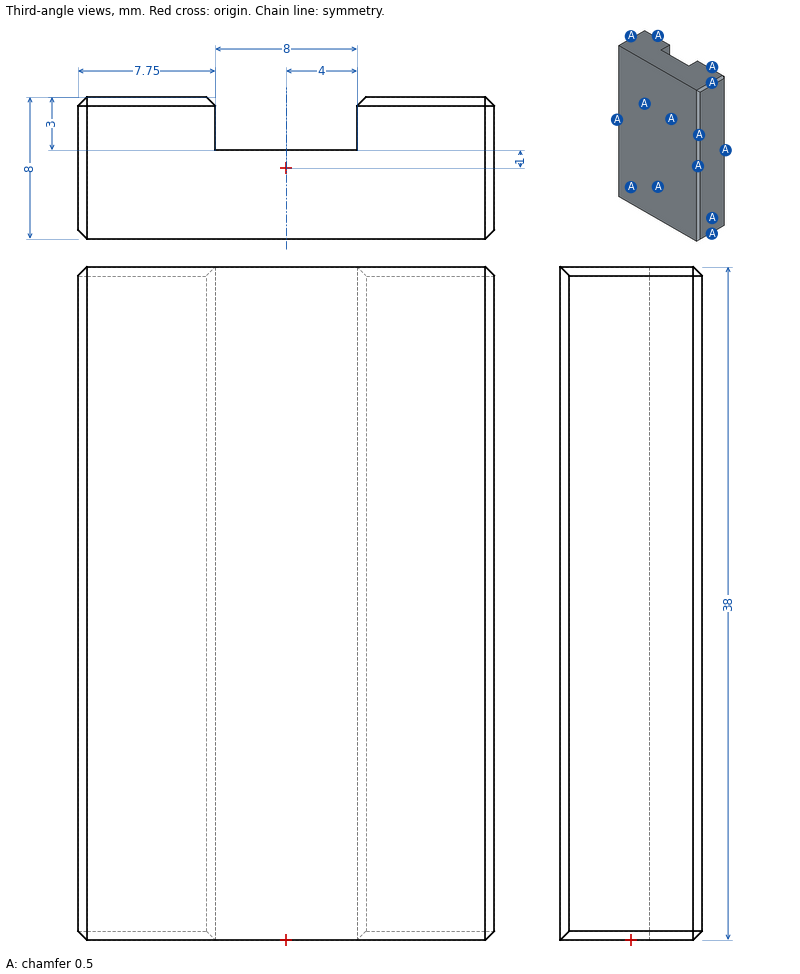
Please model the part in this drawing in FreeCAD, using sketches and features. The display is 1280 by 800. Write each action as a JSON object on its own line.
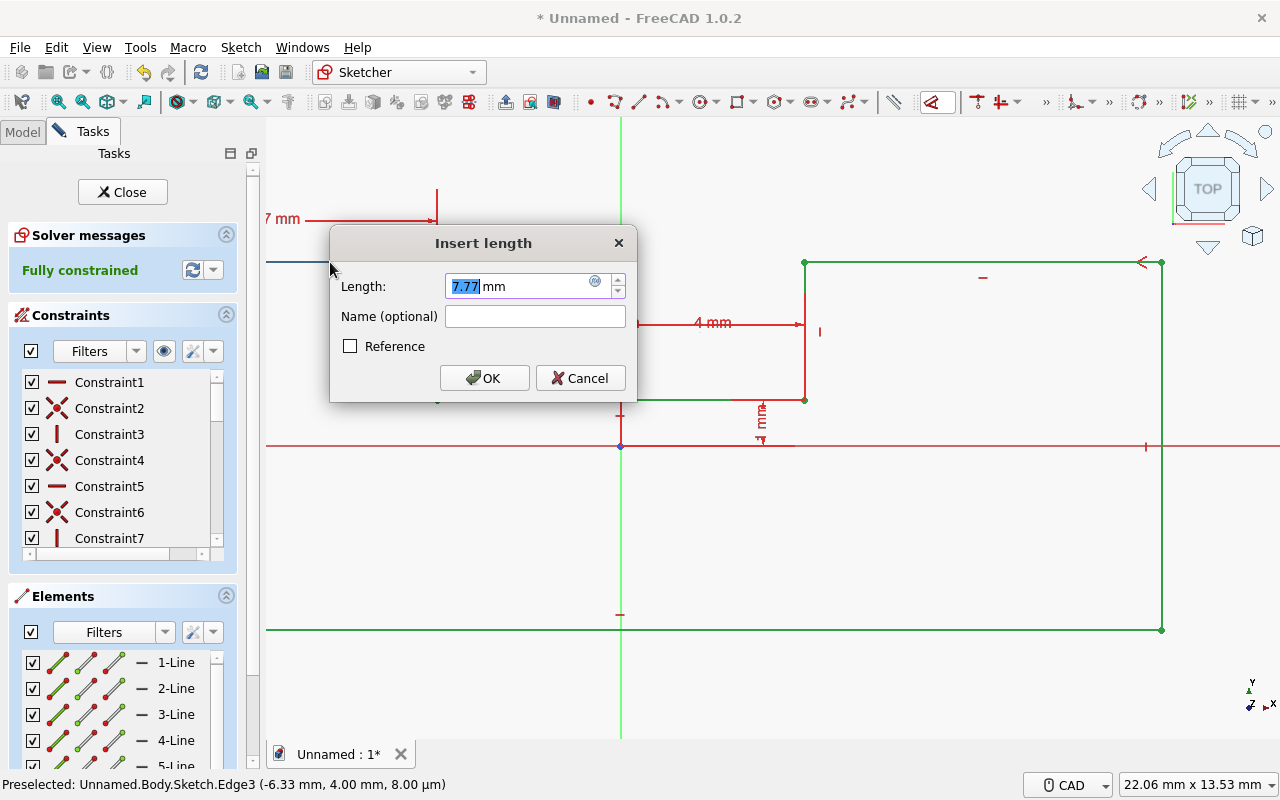
{"action": "type", "text": "7.75"}
{"action": "key", "text": "Return"}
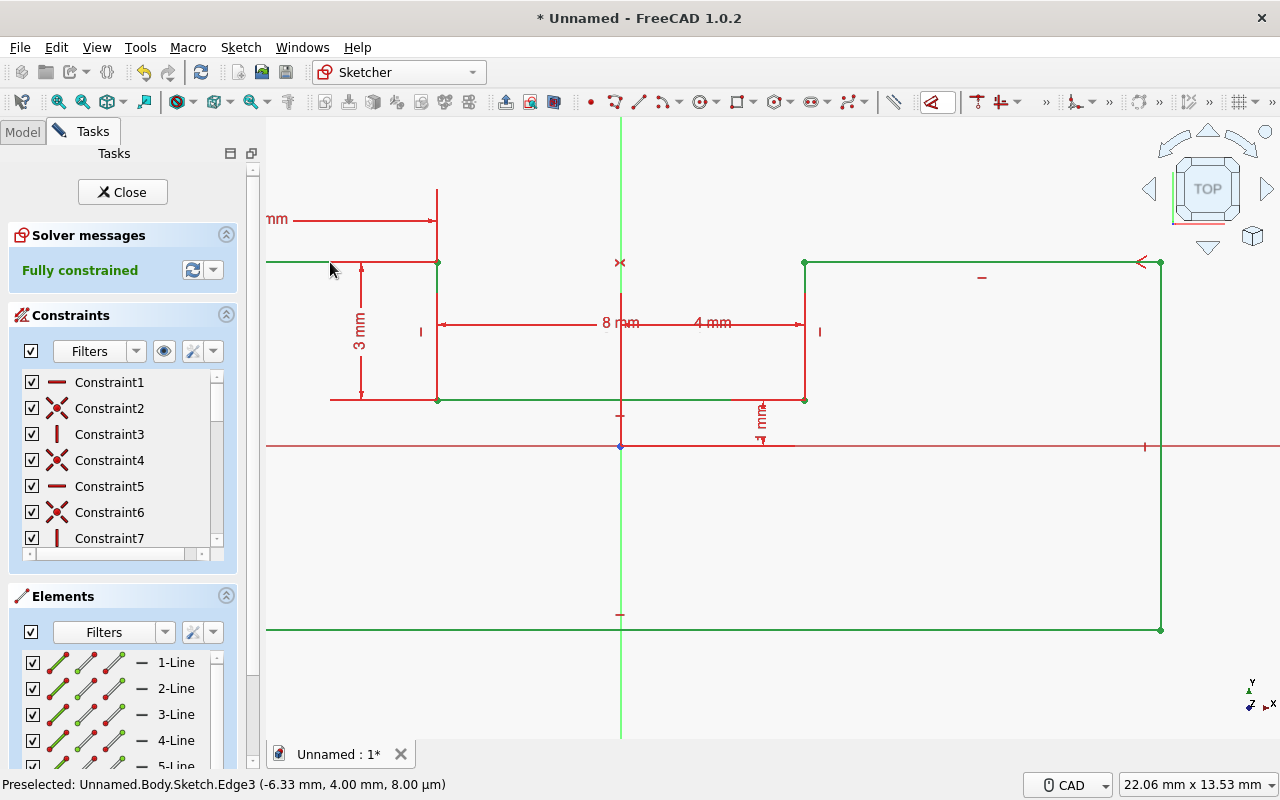
{"action": "left_click", "coordinate": [123, 192]}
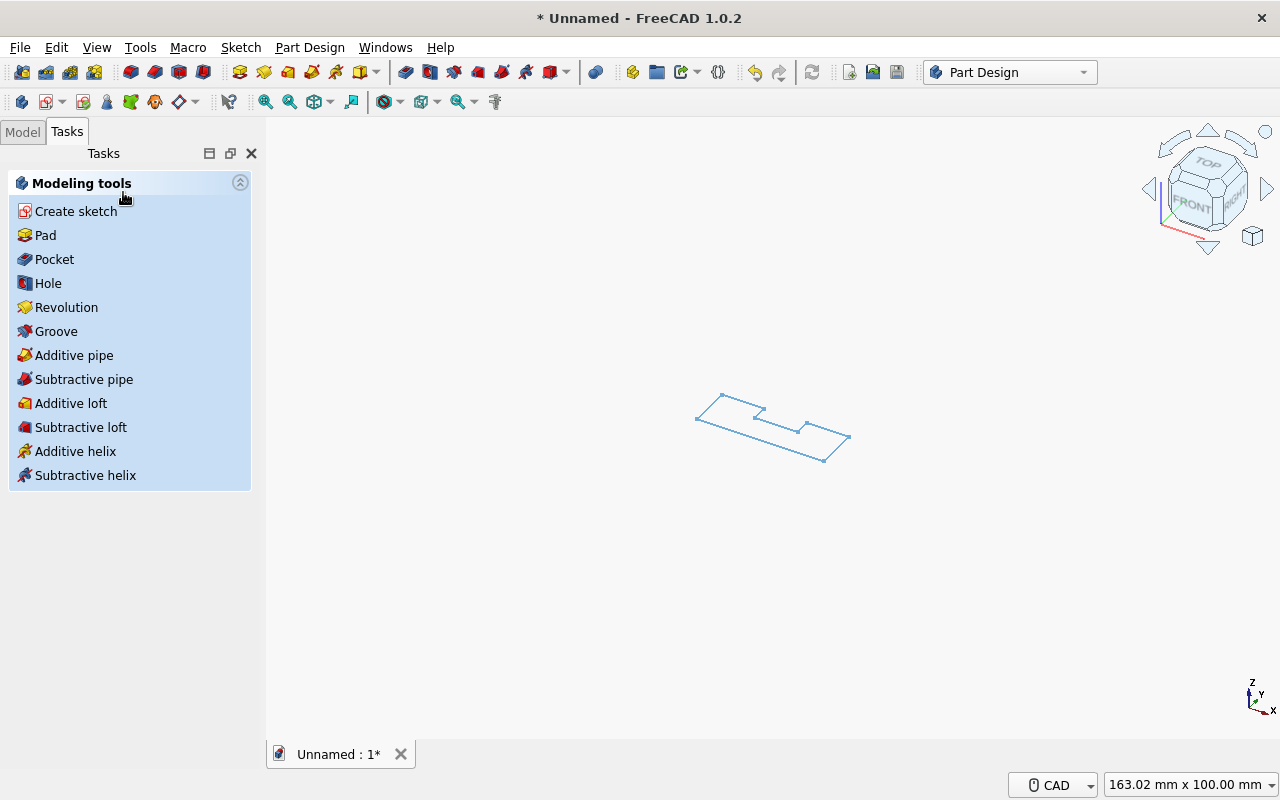
{"action": "left_click", "coordinate": [240, 72]}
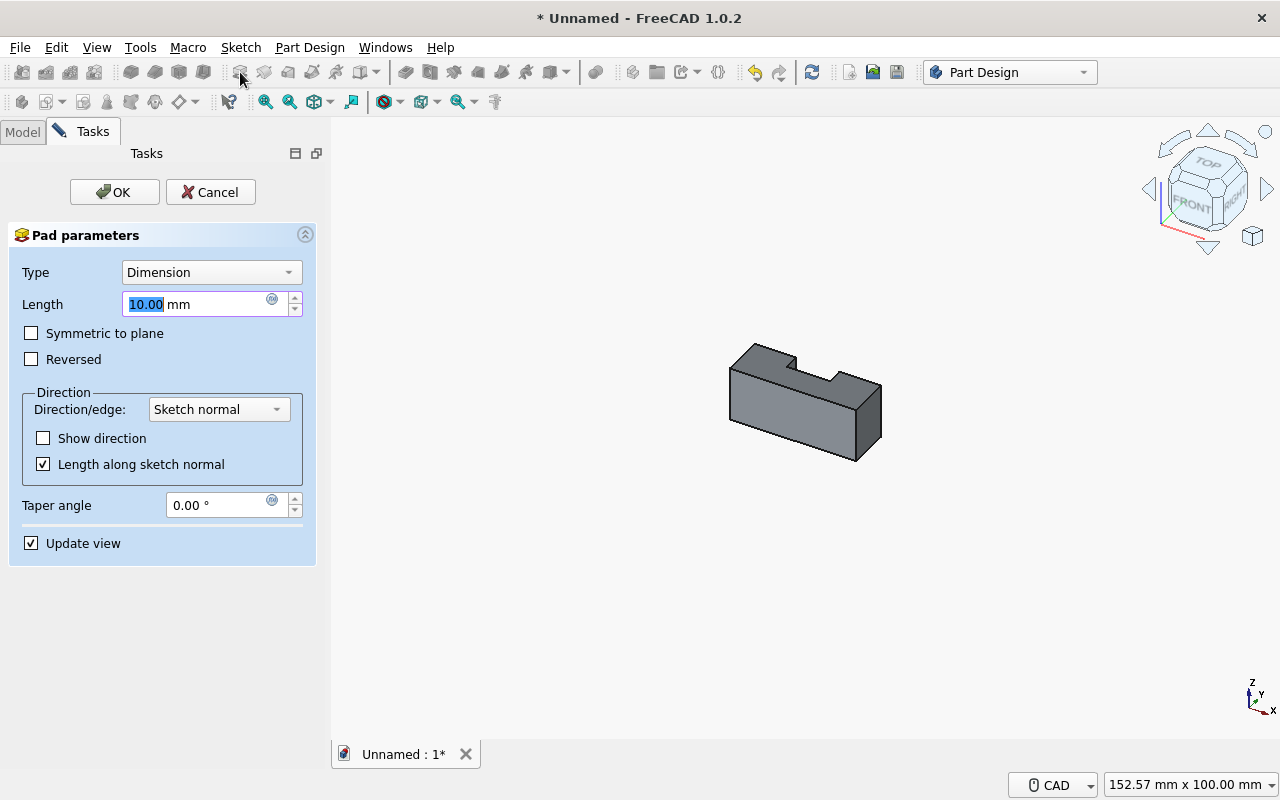
{"action": "type", "text": "38"}
{"action": "key", "text": "Tab"}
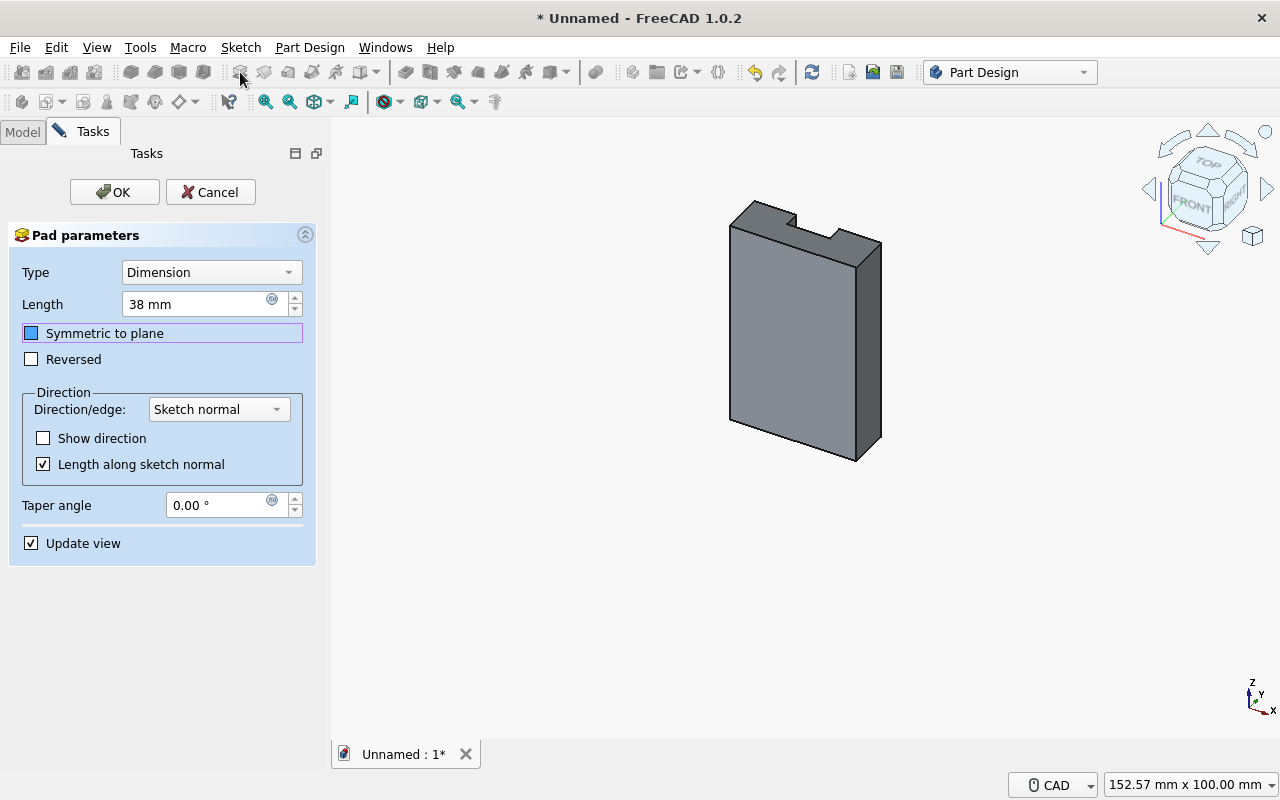
{"action": "left_click", "coordinate": [115, 192]}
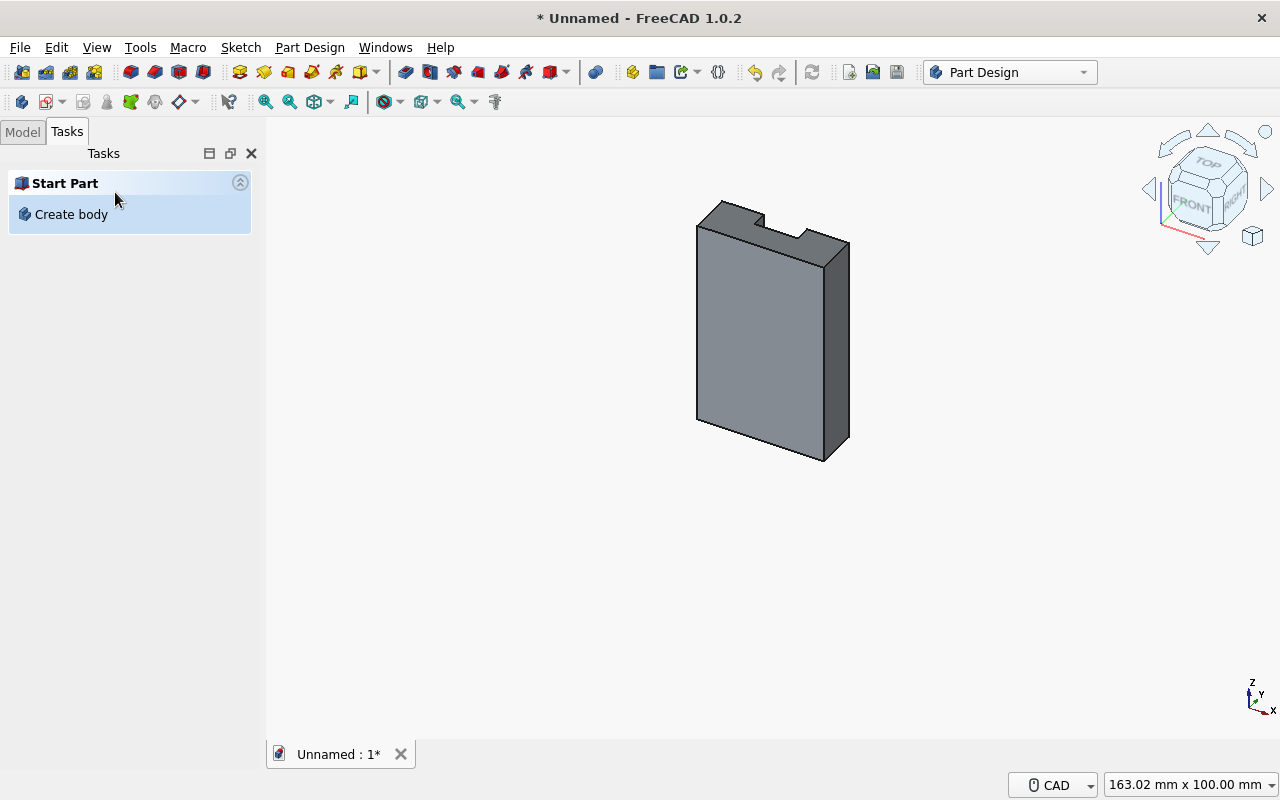
{"action": "left_click", "coordinate": [266, 102]}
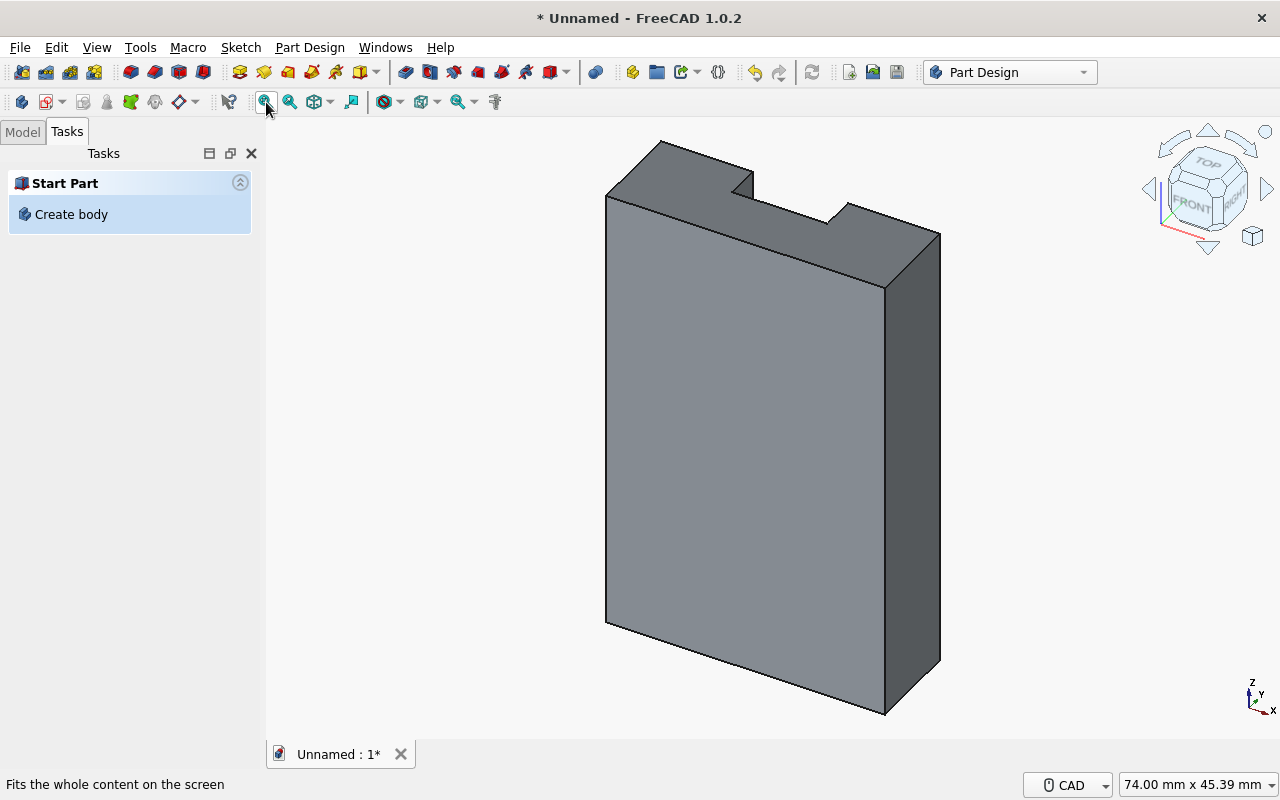
{"action": "left_click", "coordinate": [912, 351]}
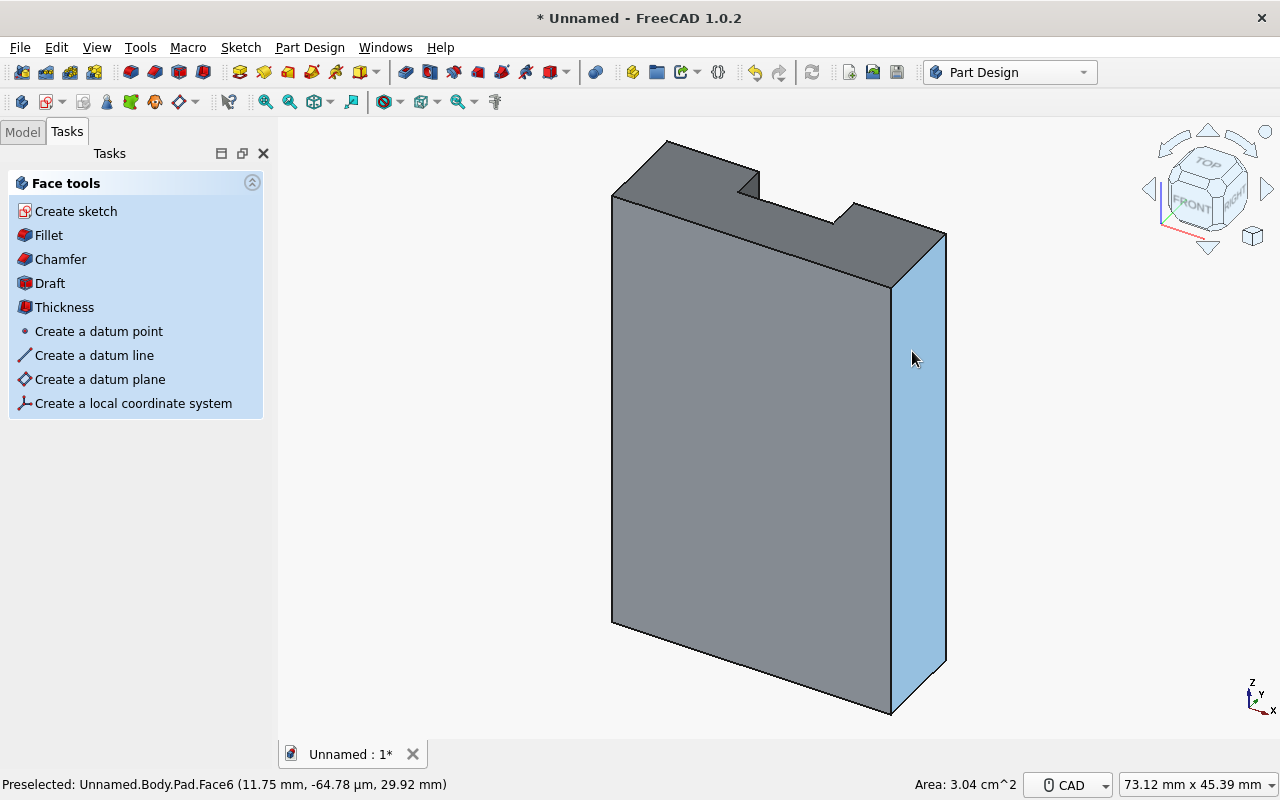
{"action": "key", "text": "0"}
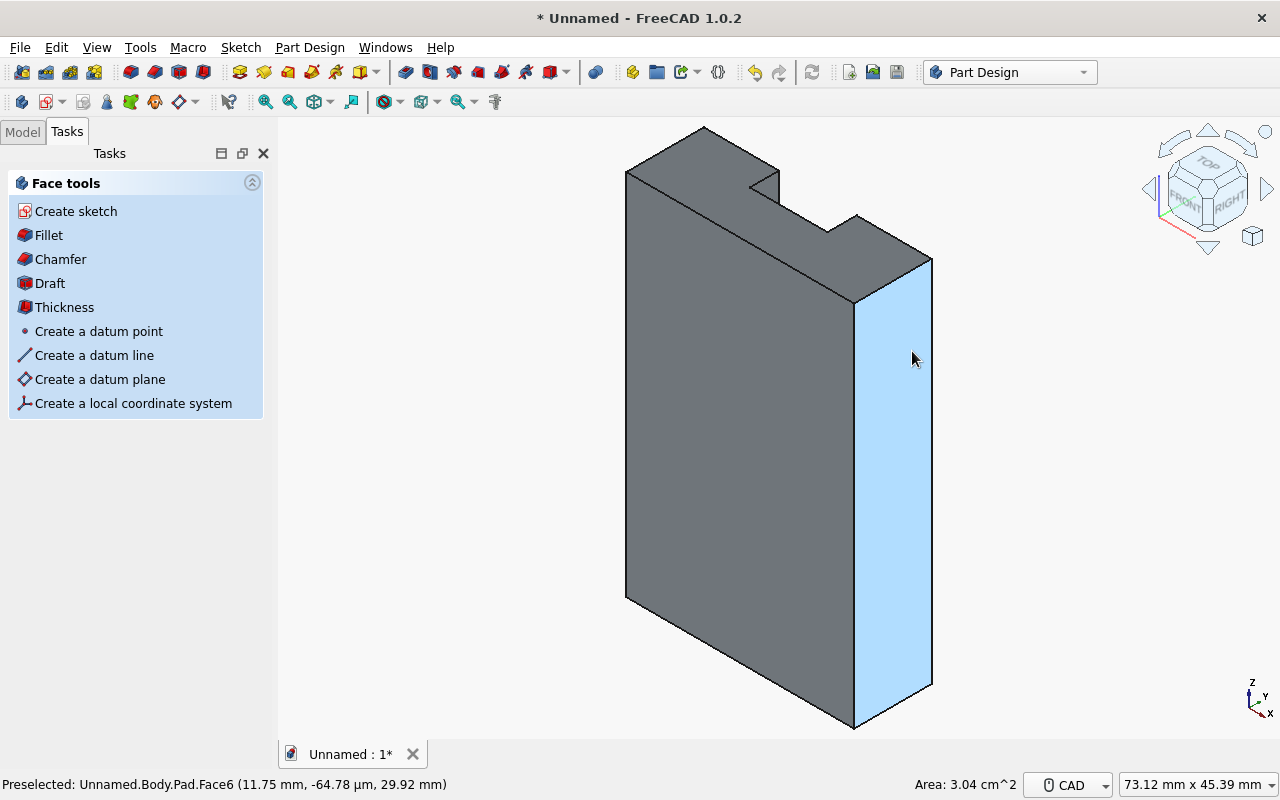
{"action": "key", "text": "2"}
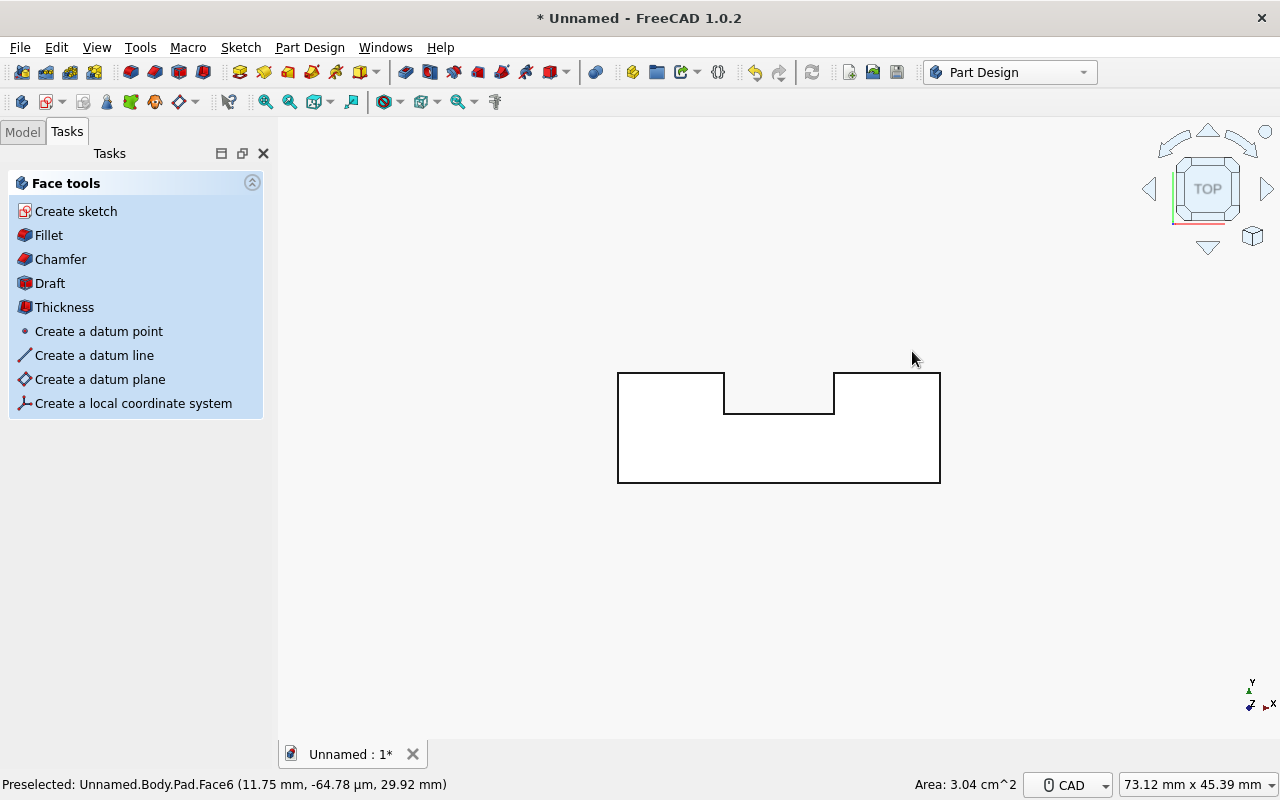
{"action": "key", "text": "v f"}